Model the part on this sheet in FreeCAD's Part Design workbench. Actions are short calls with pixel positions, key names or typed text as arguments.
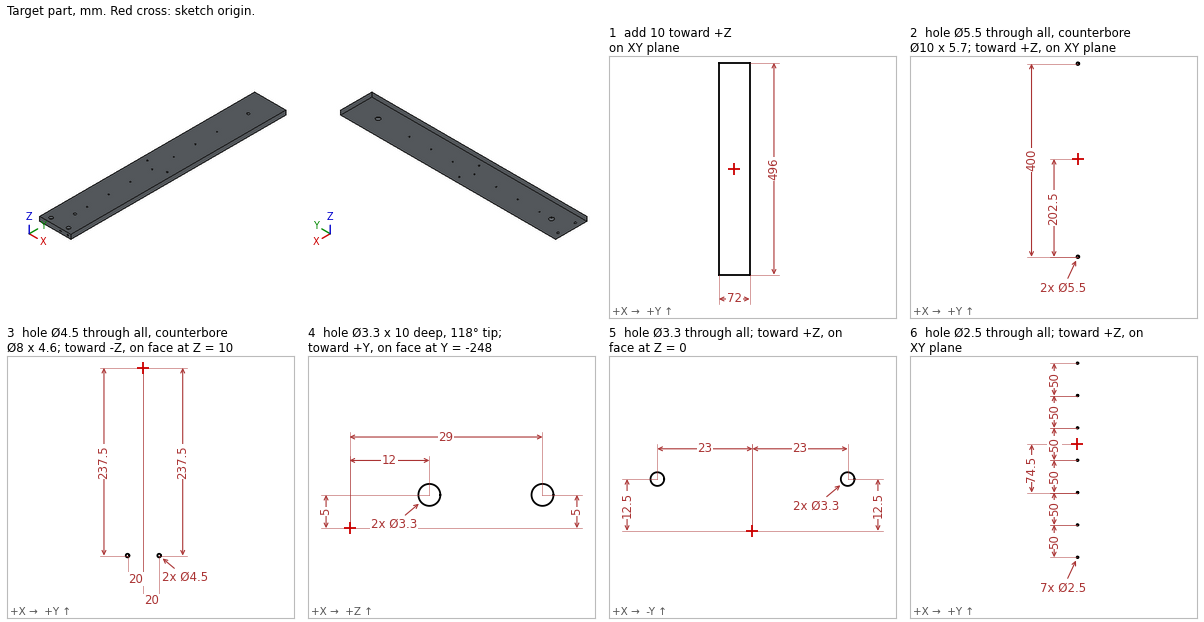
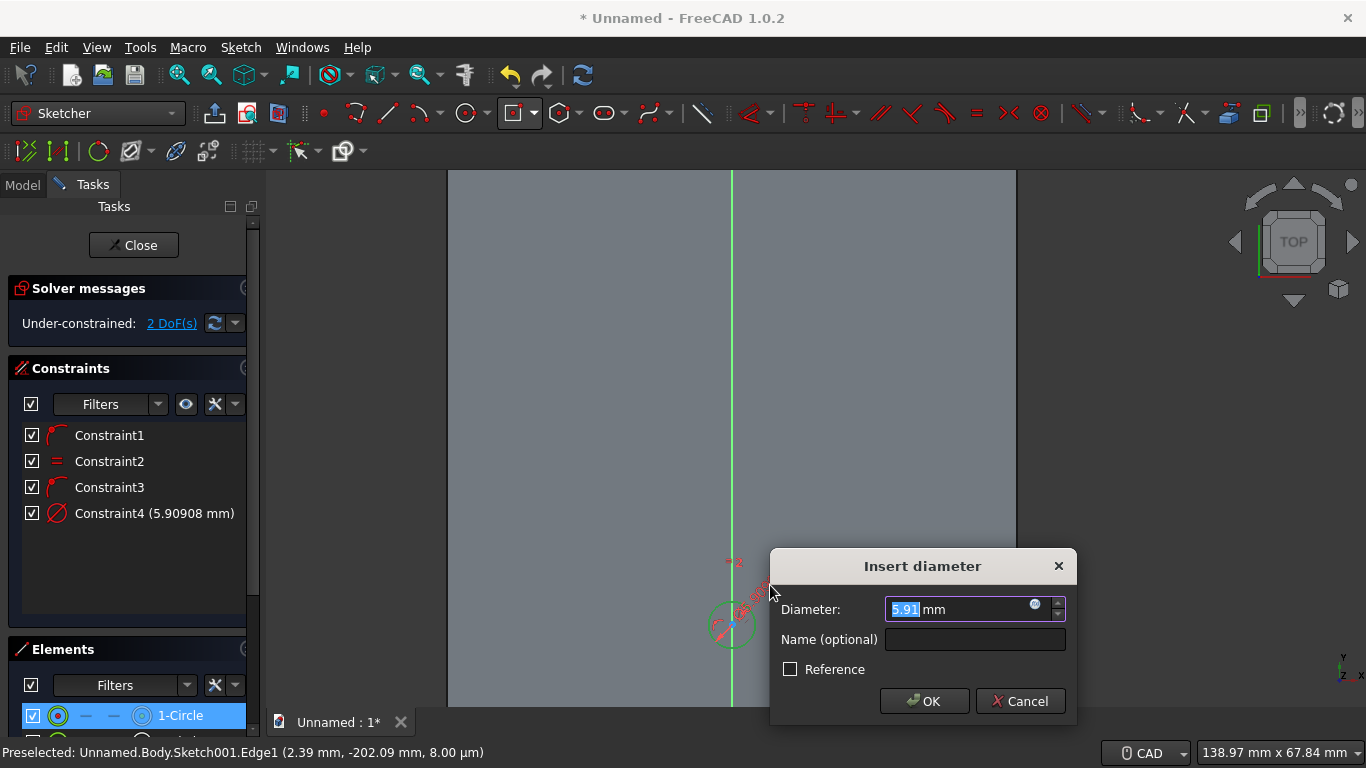
text(5.5)
key(Return)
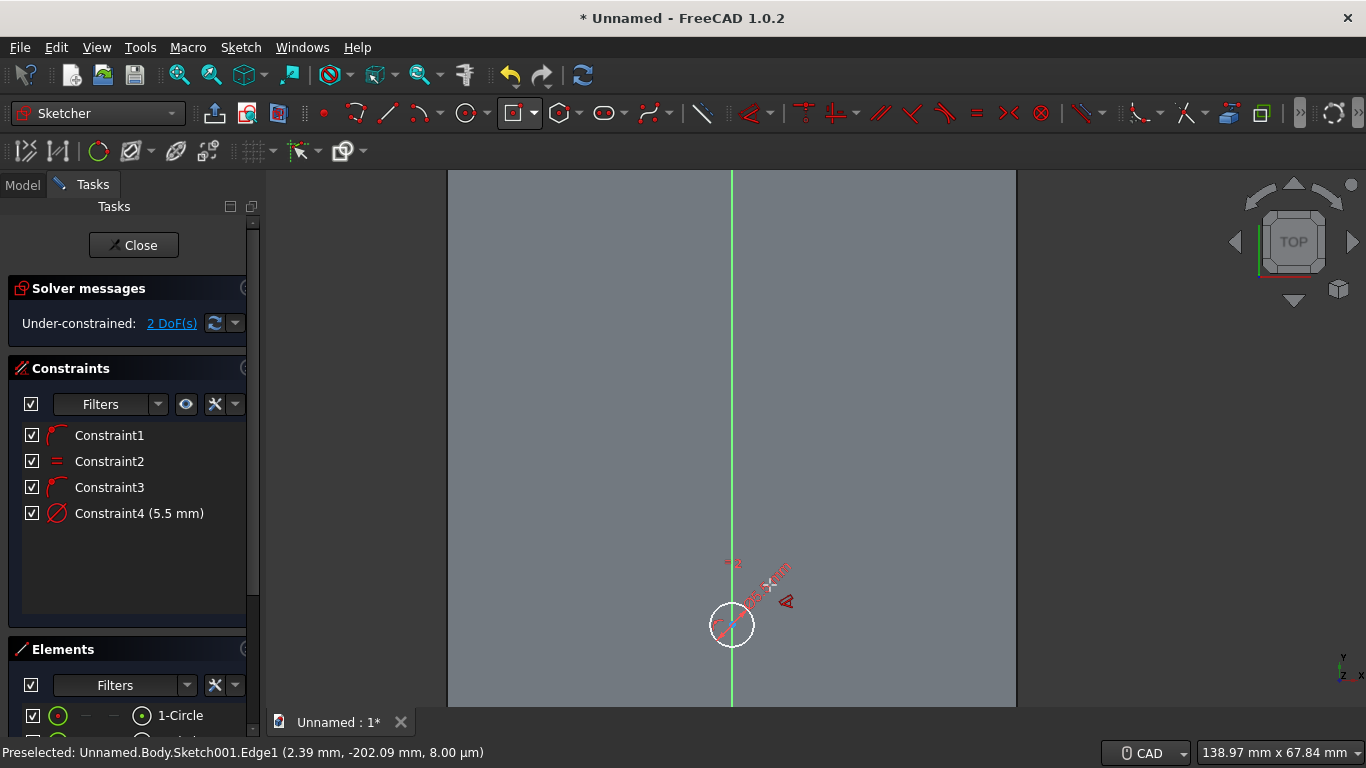
scroll(749, 614, down, 11)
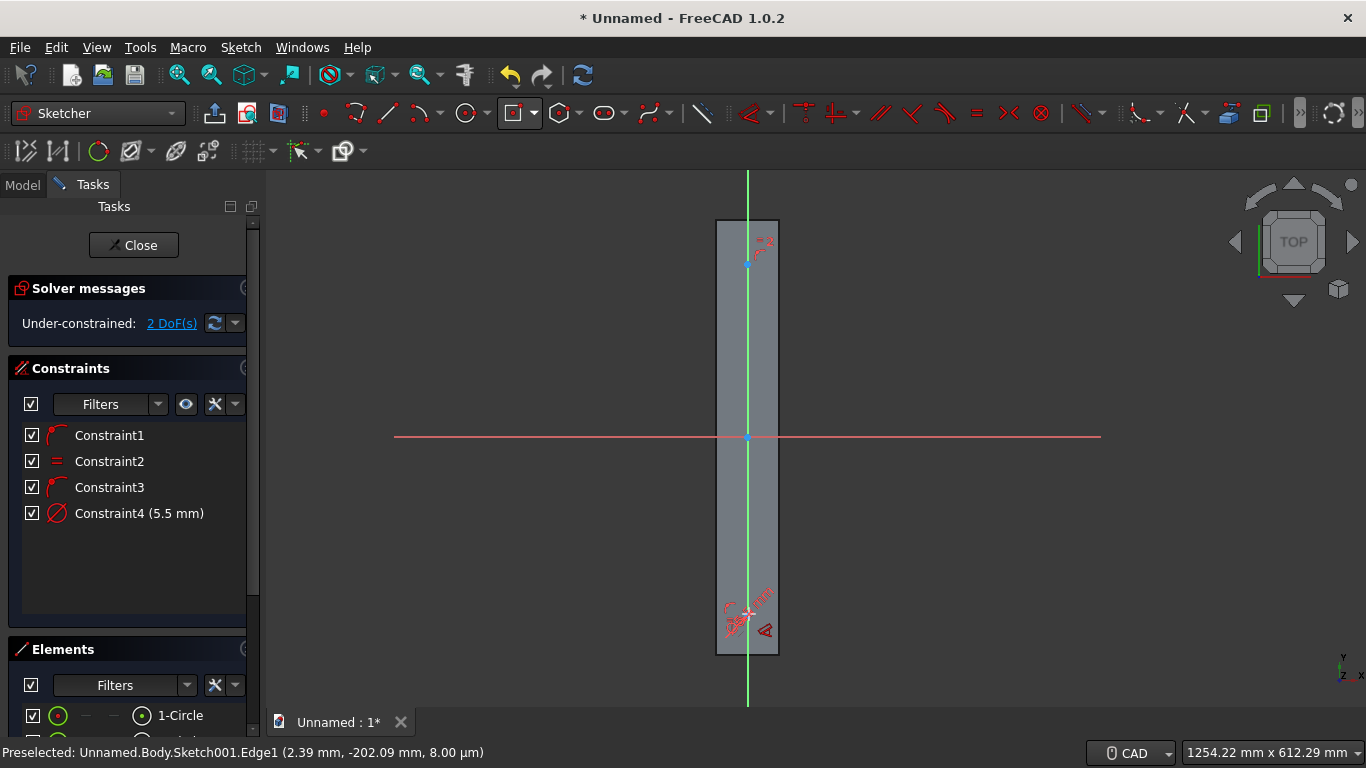
click(748, 616)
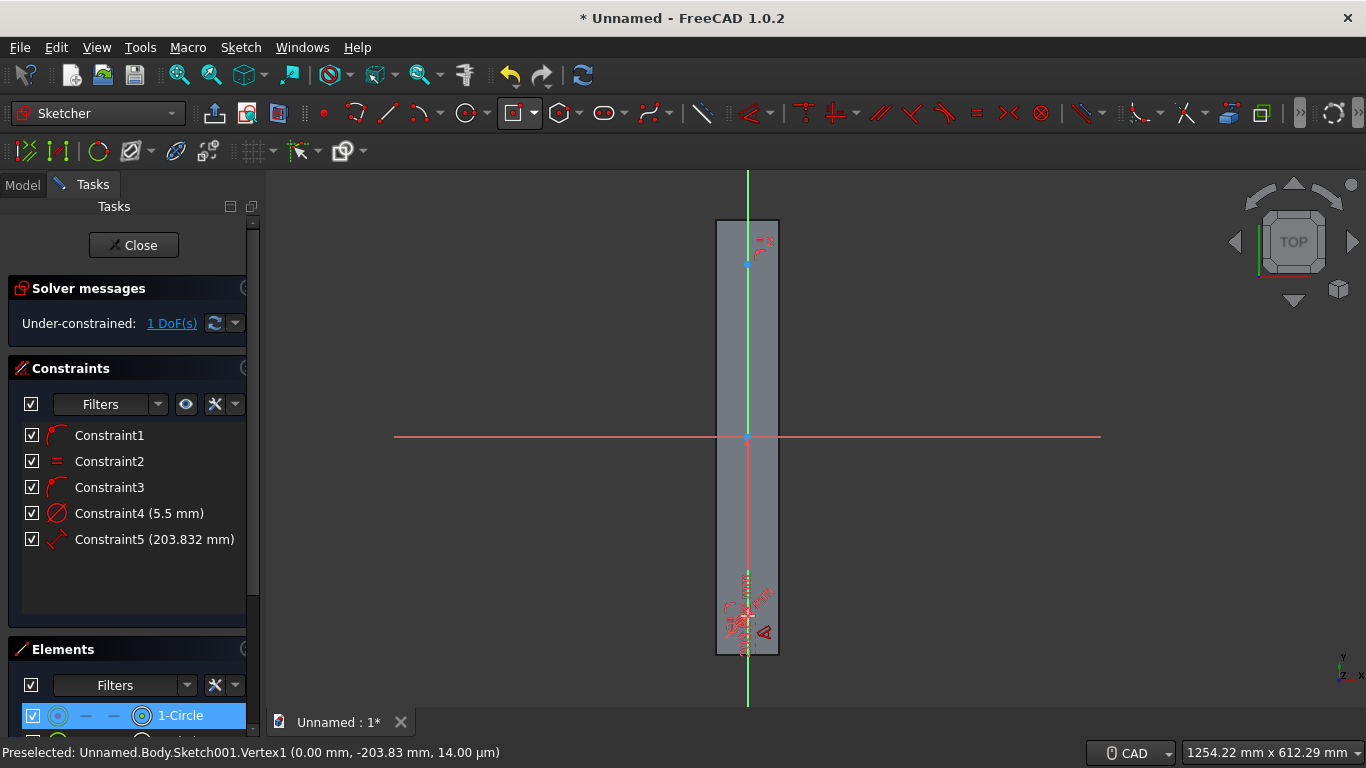
click(748, 265)
click(782, 360)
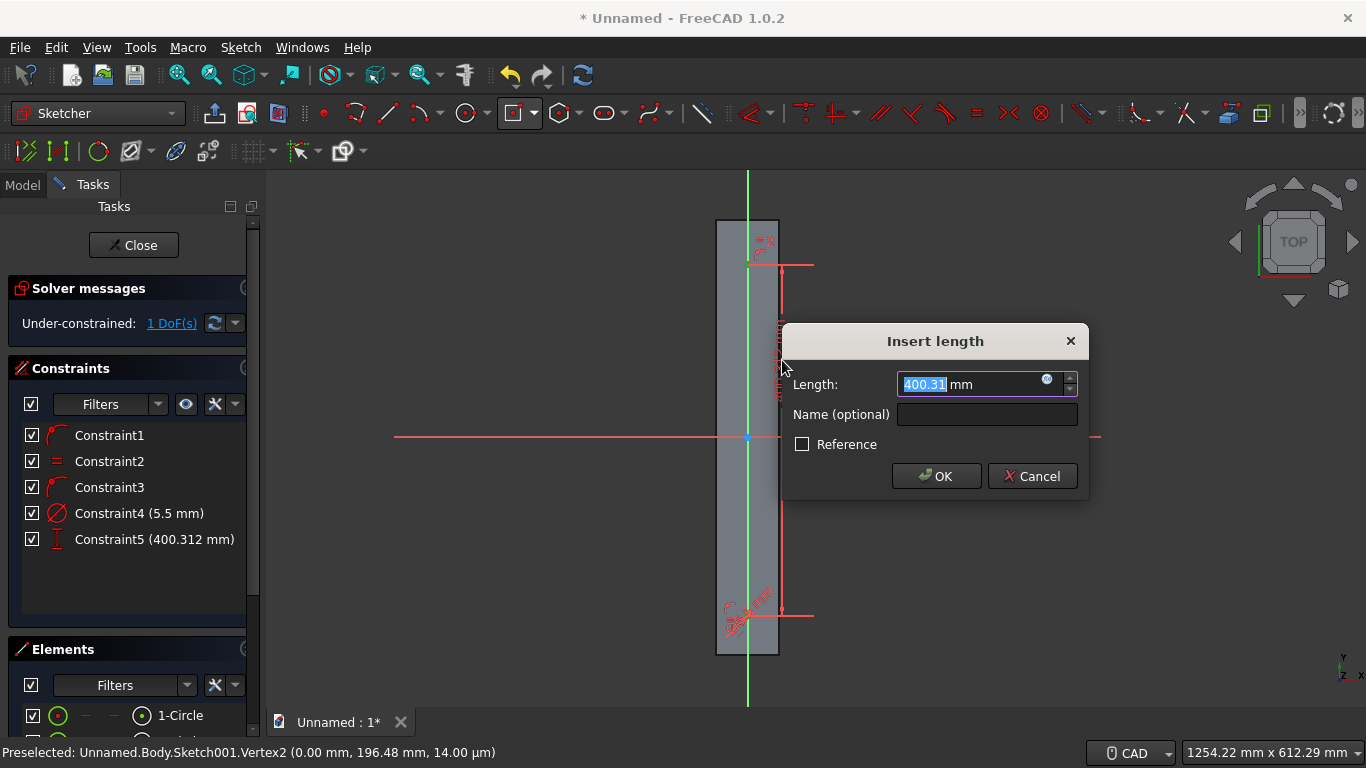
text(400)
key(Return)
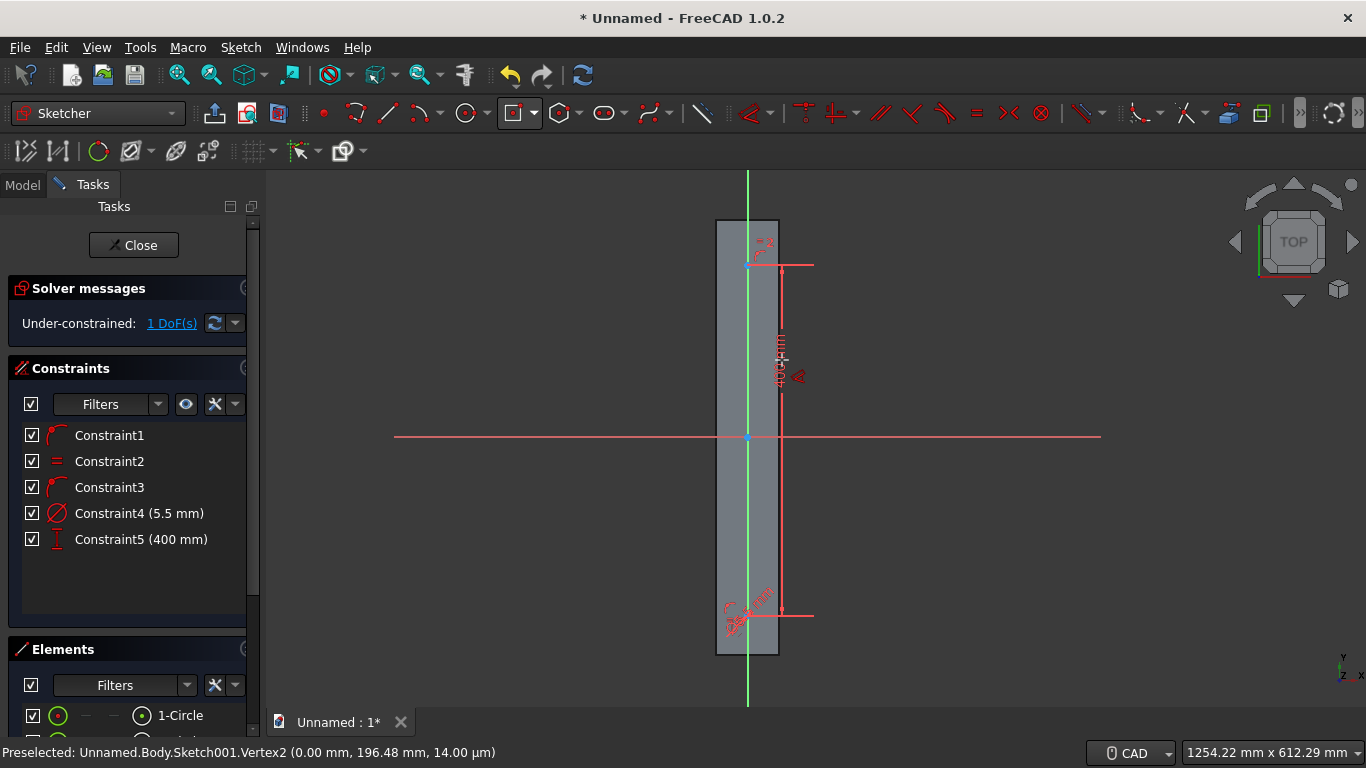
click(748, 616)
click(782, 527)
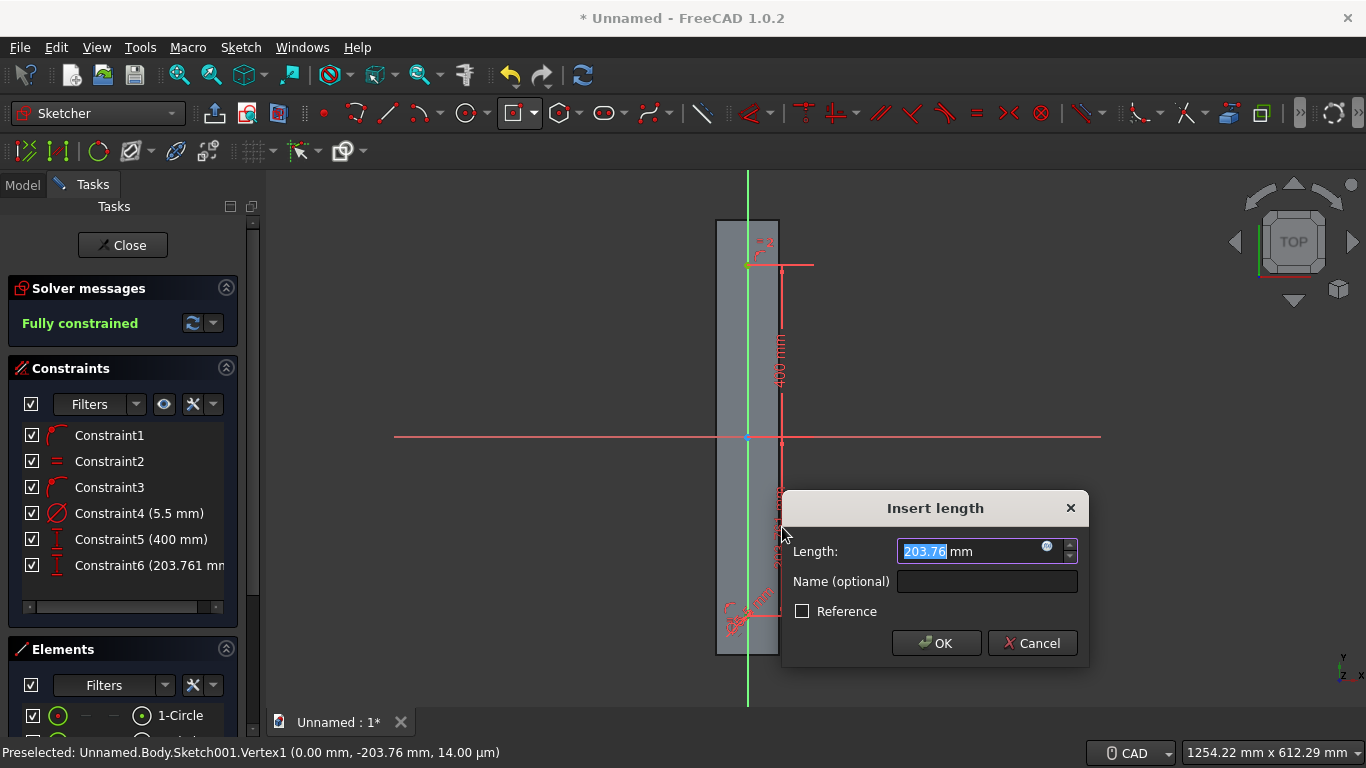
text(202.5)
key(Return)
key(Escape)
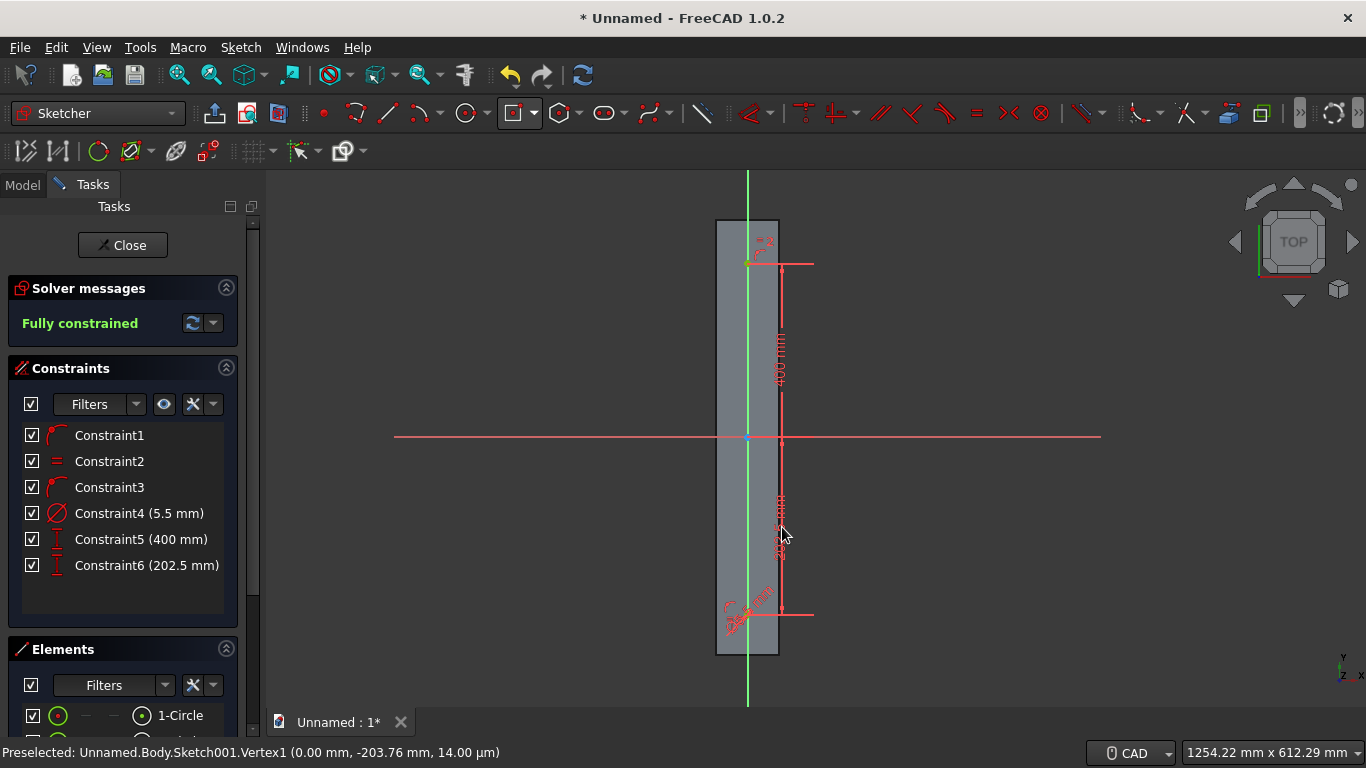
click(123, 245)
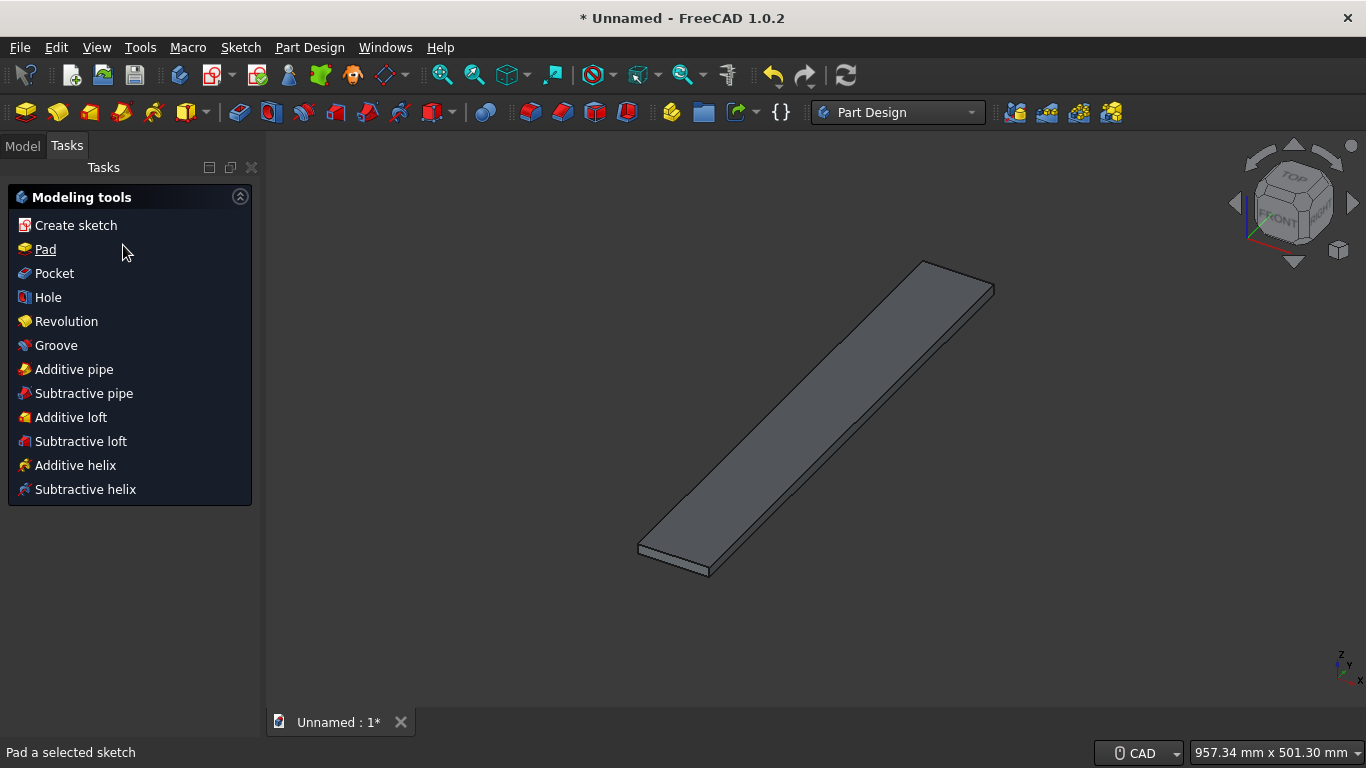
click(272, 112)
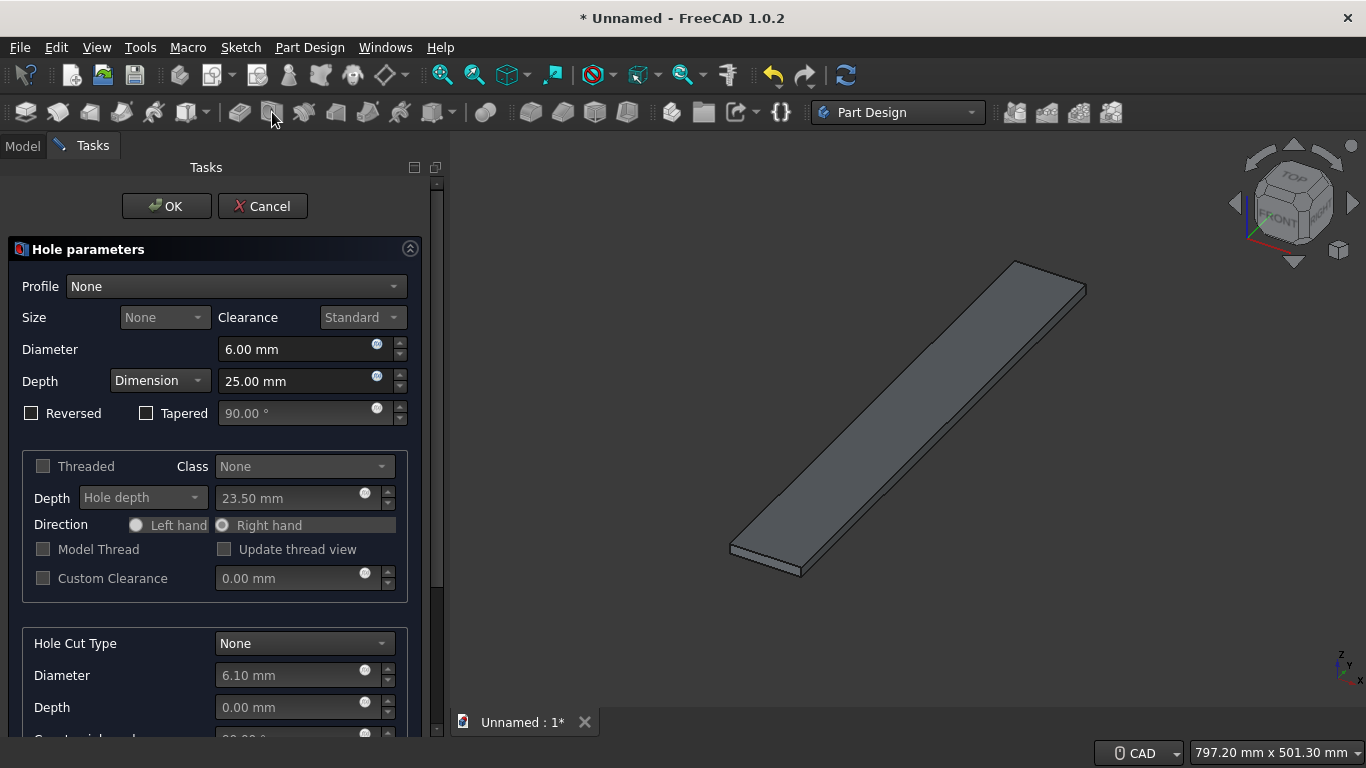
triple_click(305, 349)